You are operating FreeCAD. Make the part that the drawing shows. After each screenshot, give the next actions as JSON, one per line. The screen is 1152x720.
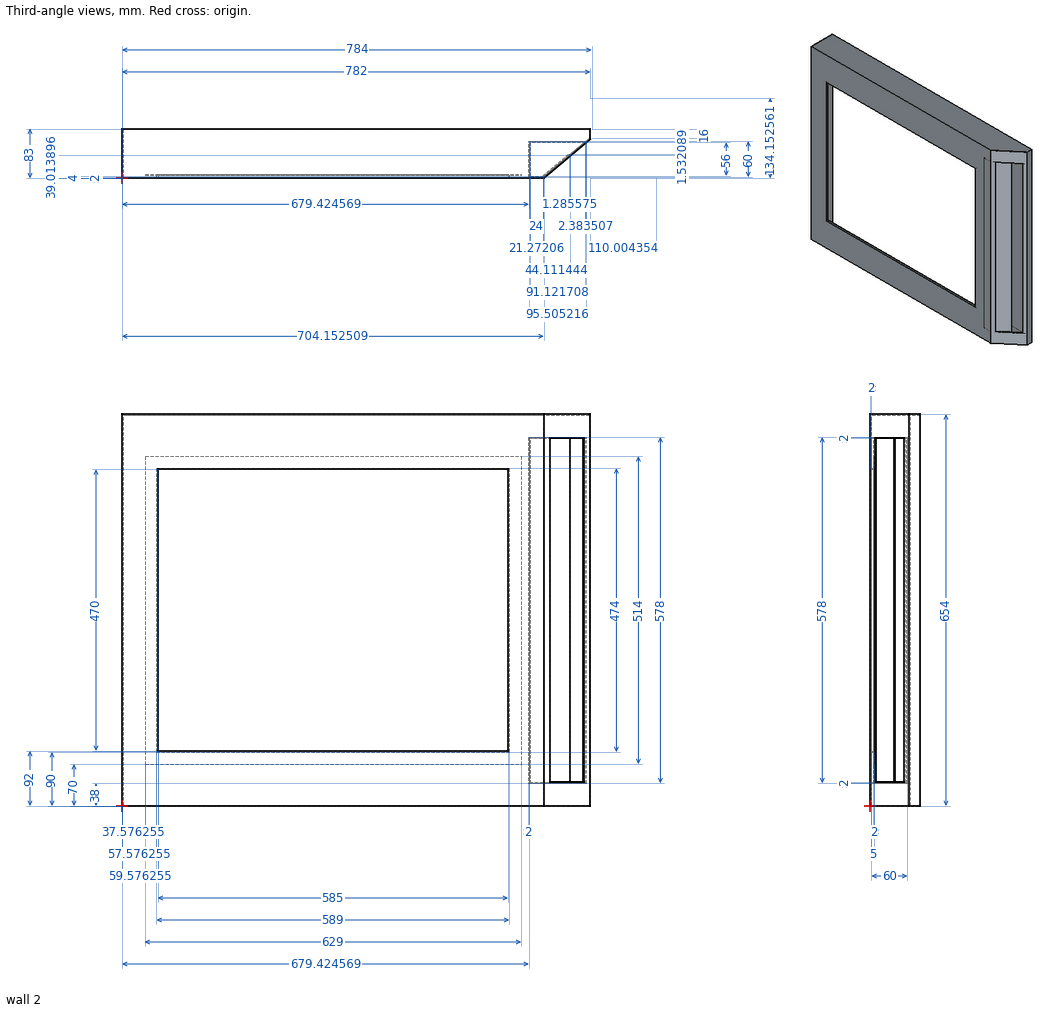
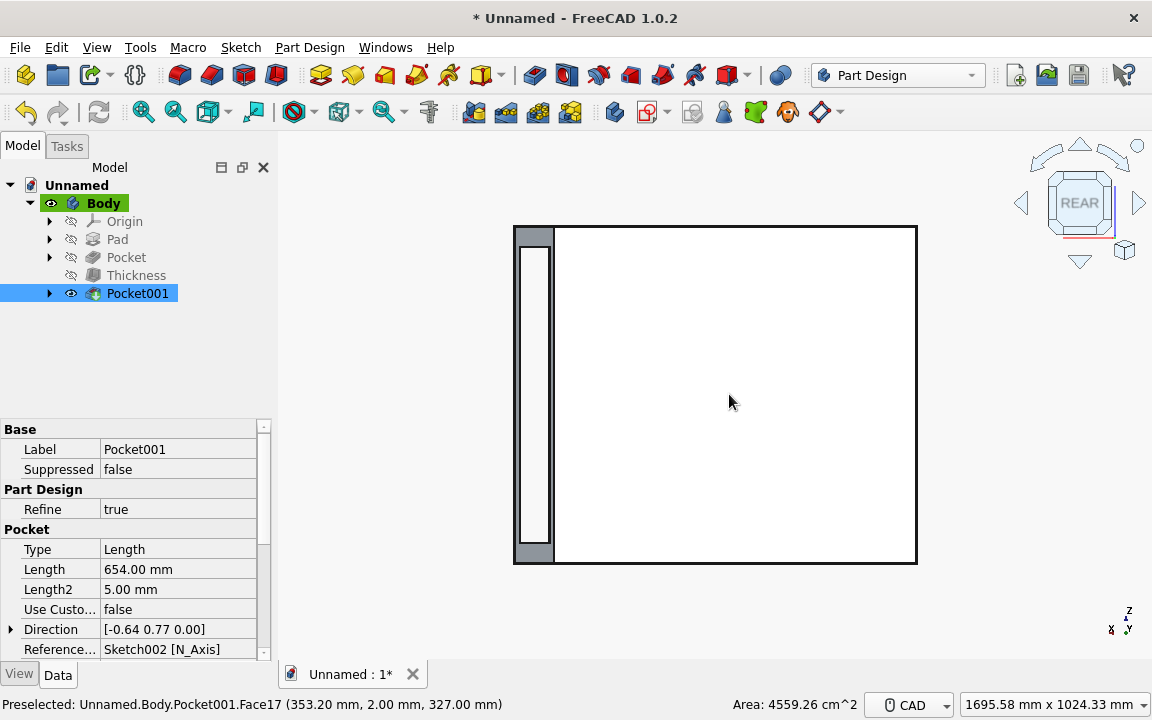
{"action": "left_click", "coordinate": [648, 112]}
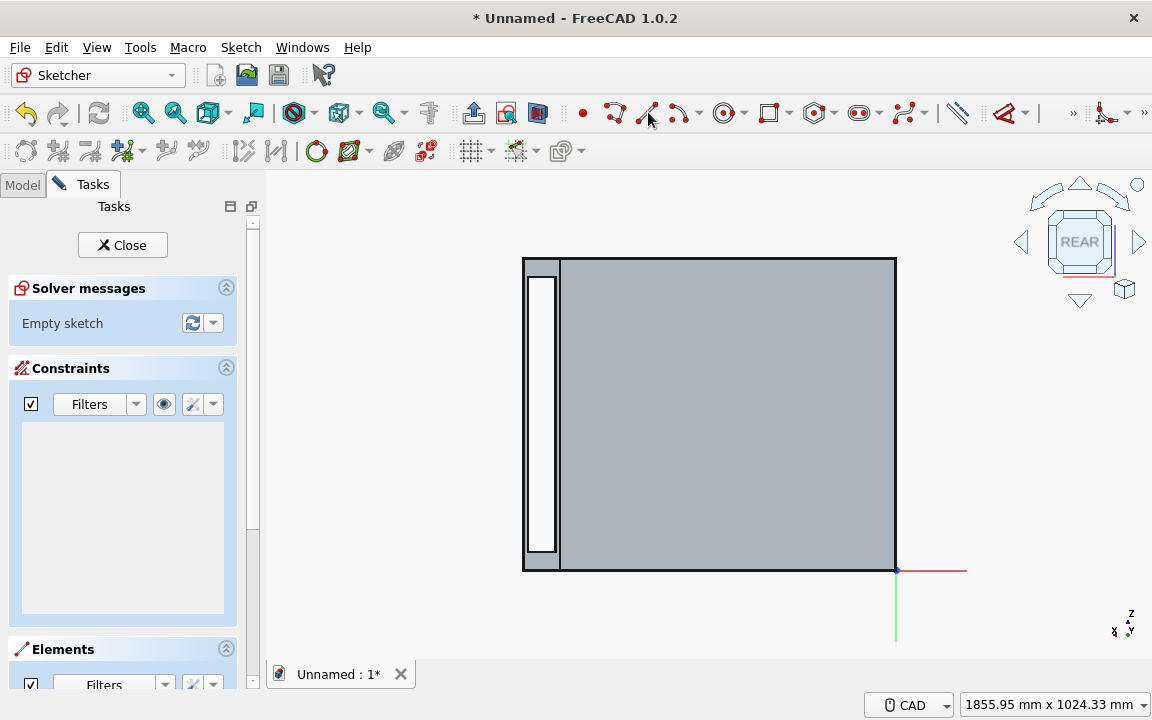
{"action": "key", "text": "q s"}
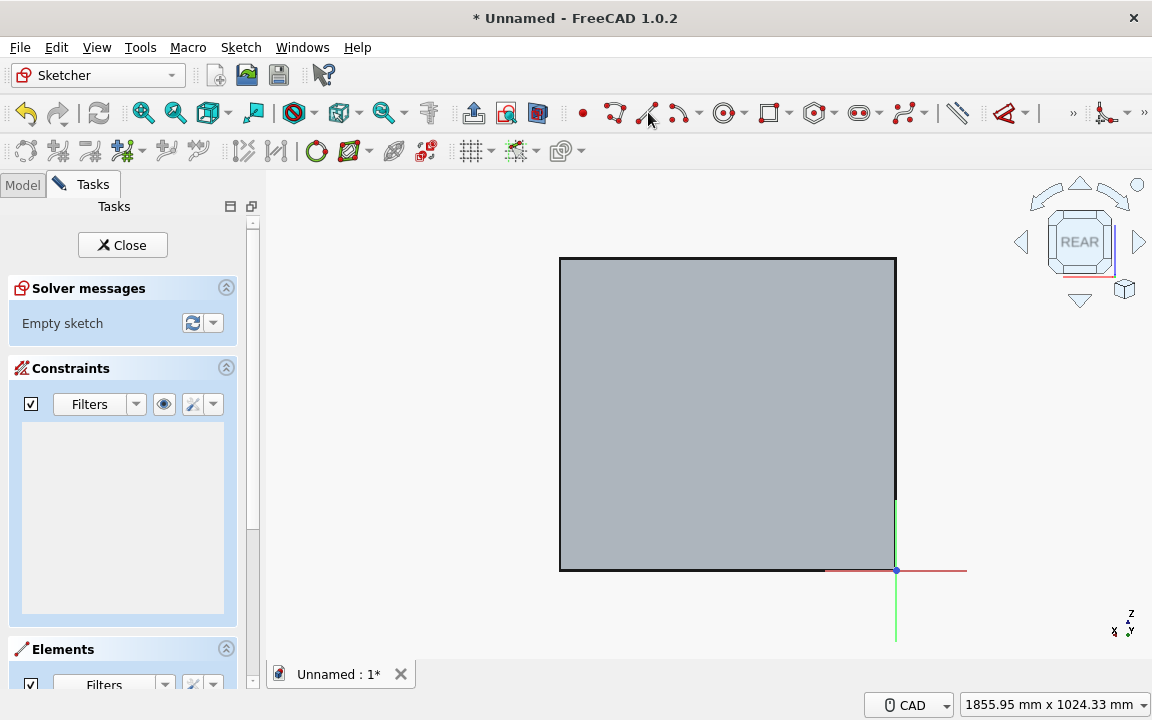
{"action": "key", "text": "g r"}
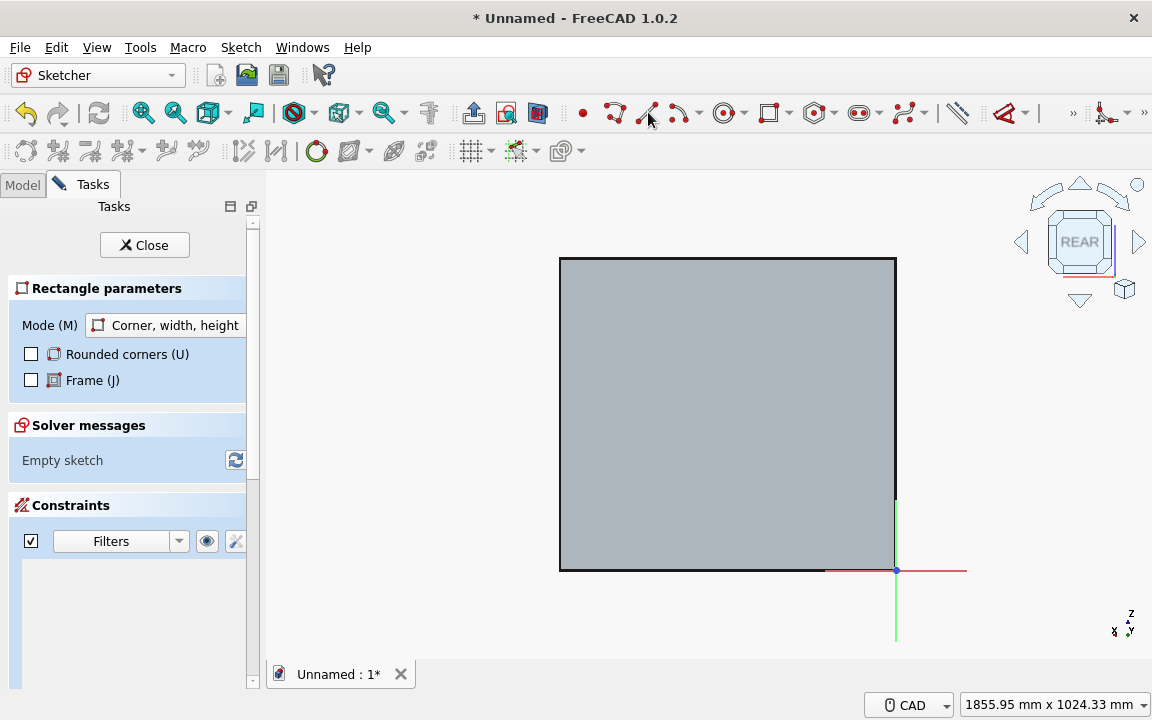
{"action": "scroll", "coordinate": [572, 277], "scroll_direction": "up", "scroll_amount": 15}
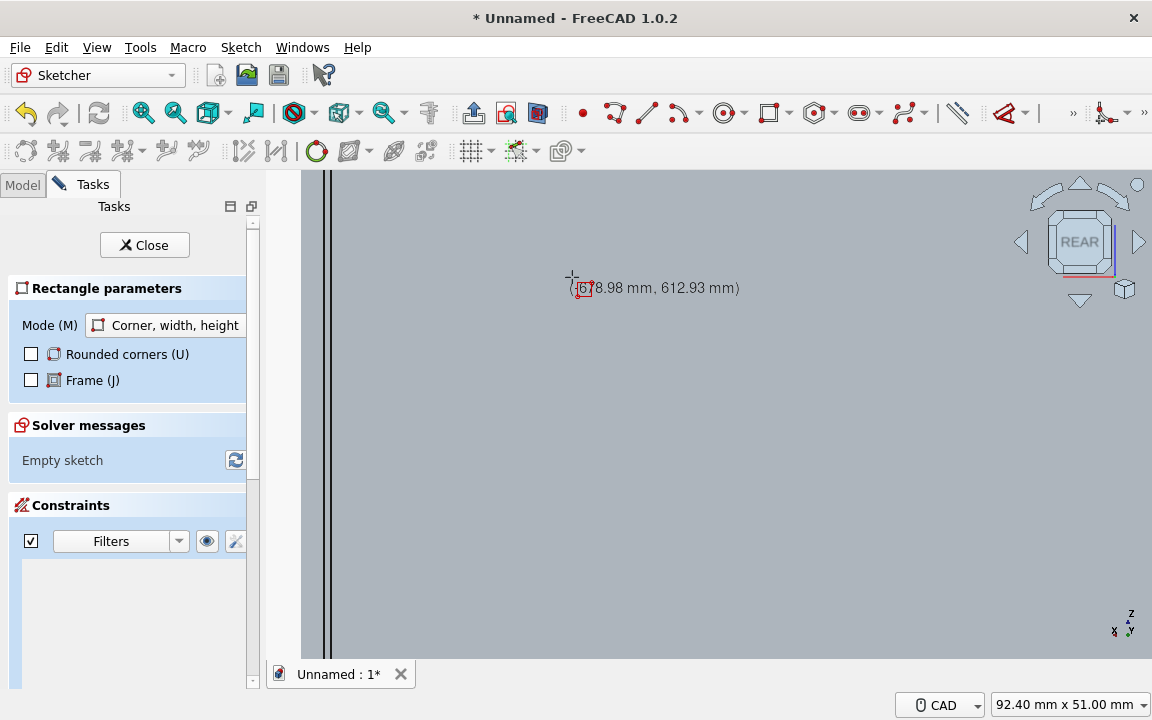
{"action": "scroll", "coordinate": [474, 268], "scroll_direction": "down", "scroll_amount": 15}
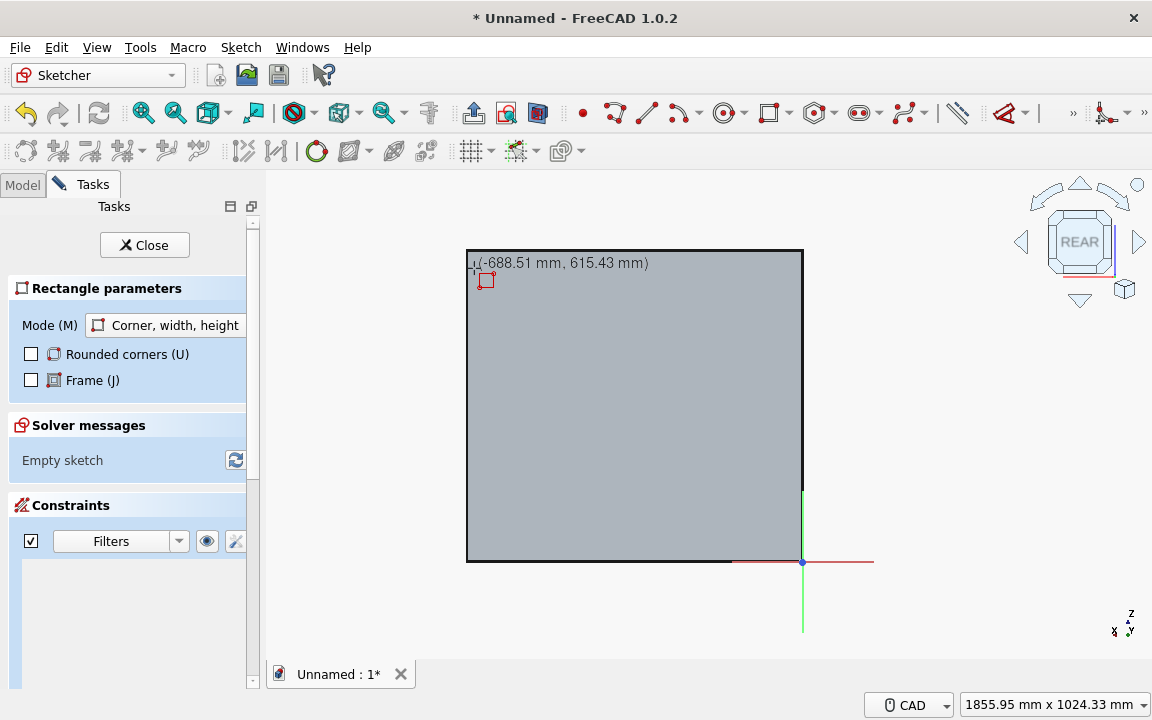
{"action": "left_click", "coordinate": [479, 268]}
{"action": "left_click", "coordinate": [480, 544]}
{"action": "key", "text": "Escape"}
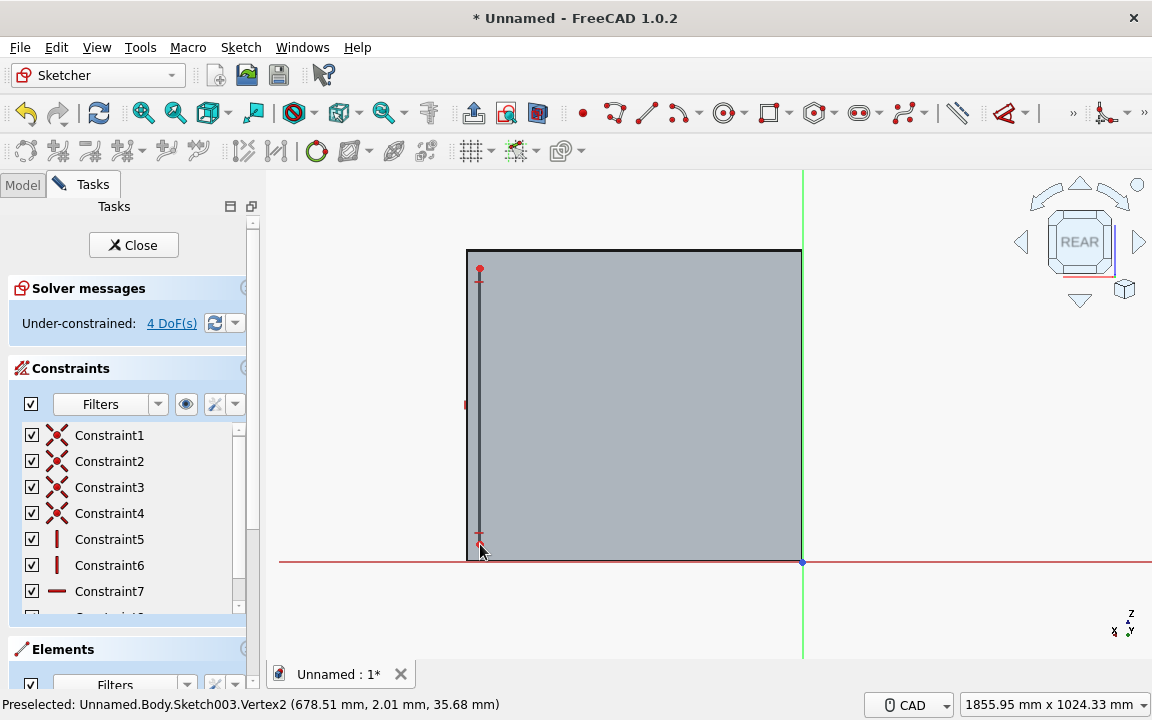
{"action": "key", "text": "d"}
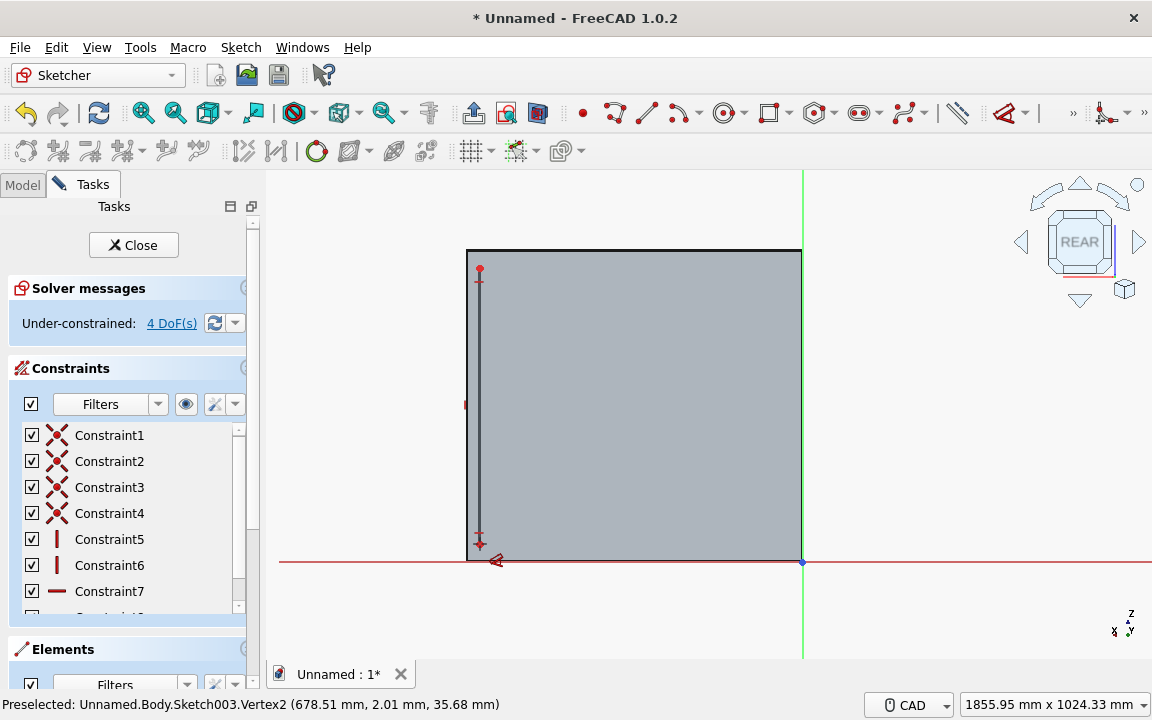
{"action": "scroll", "coordinate": [480, 545], "scroll_direction": "up", "scroll_amount": 19}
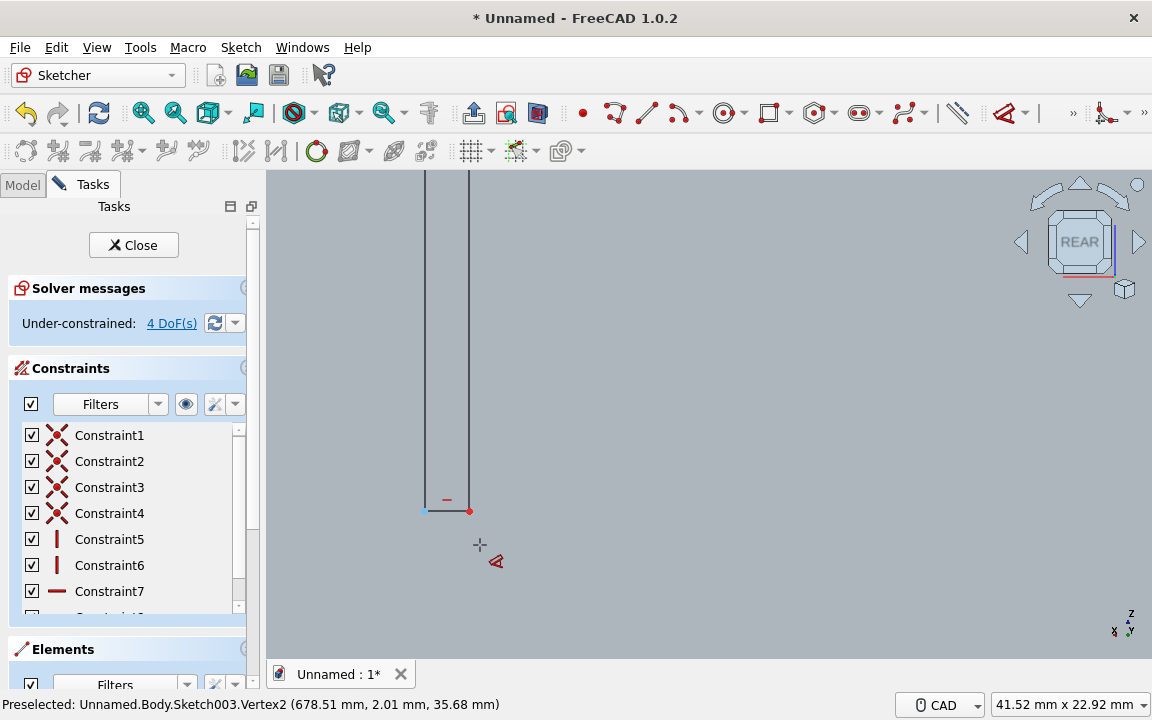
{"action": "left_click", "coordinate": [447, 511]}
{"action": "left_click", "coordinate": [447, 545]}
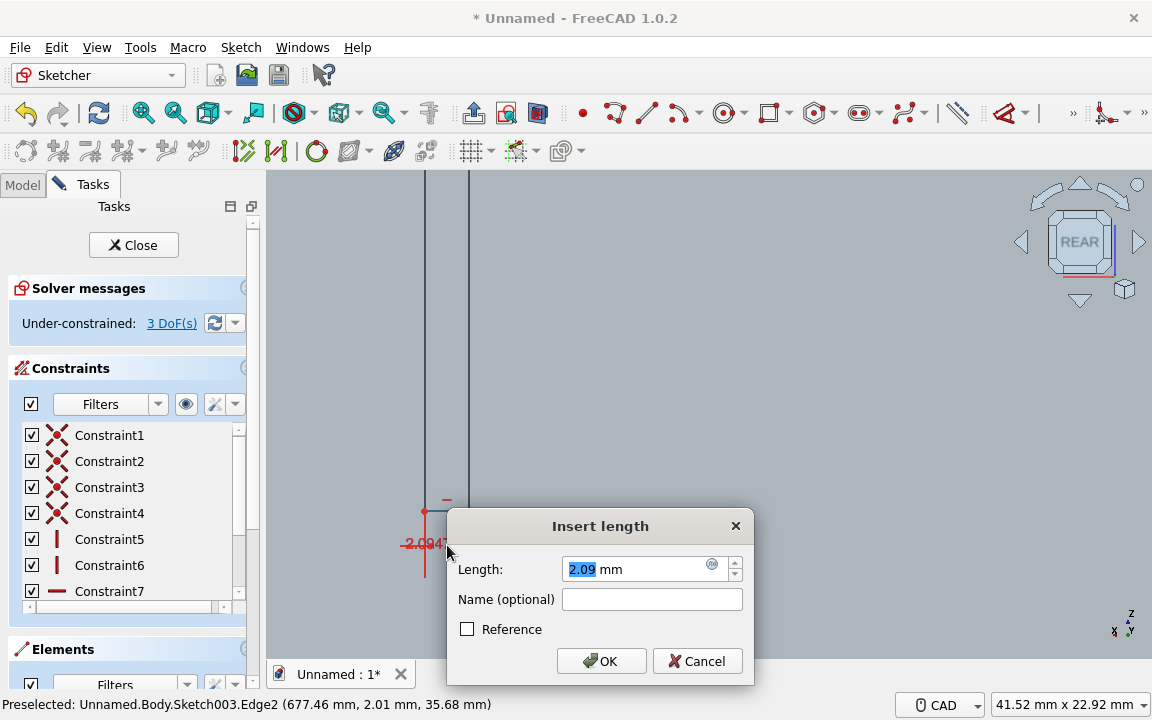
{"action": "type", "text": "2"}
{"action": "key", "text": "Return"}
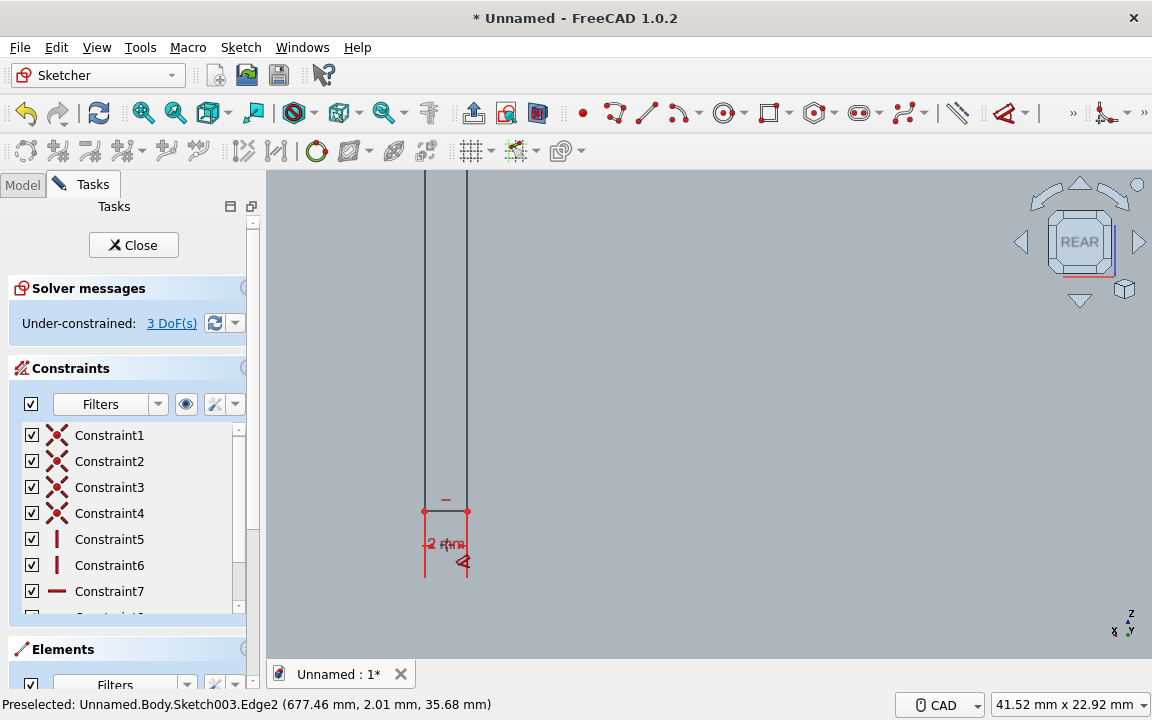
{"action": "scroll", "coordinate": [443, 575], "scroll_direction": "down", "scroll_amount": 18}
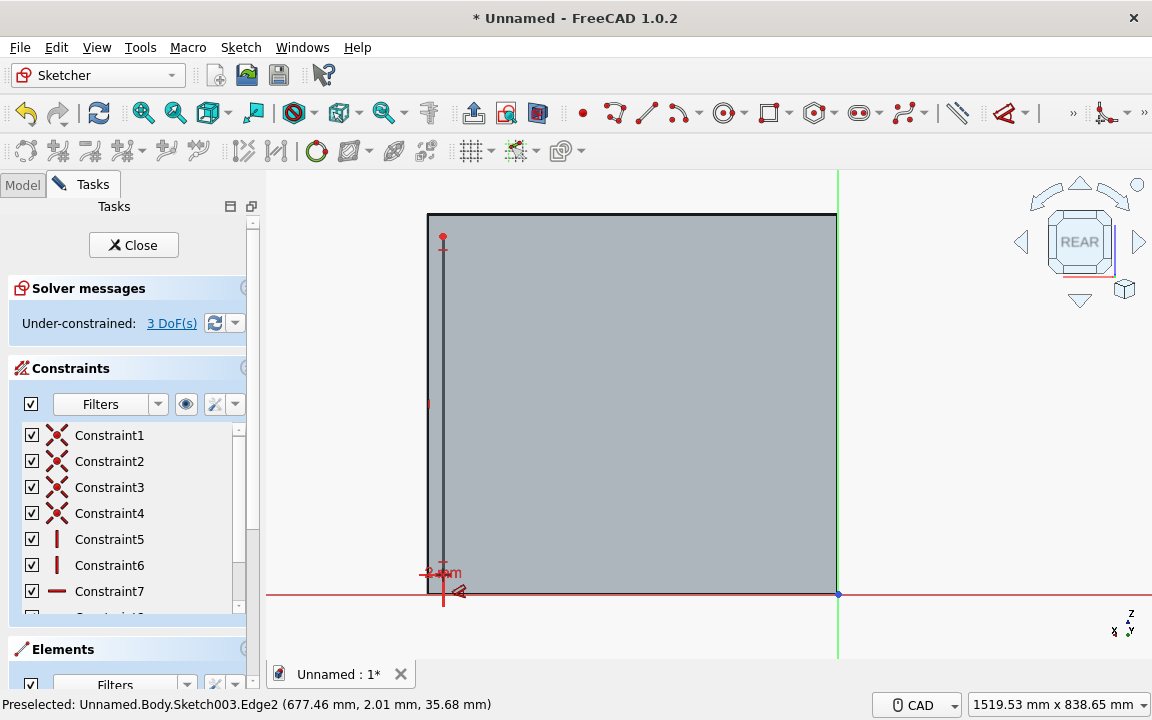
{"action": "scroll", "coordinate": [443, 338], "scroll_direction": "up", "scroll_amount": 13}